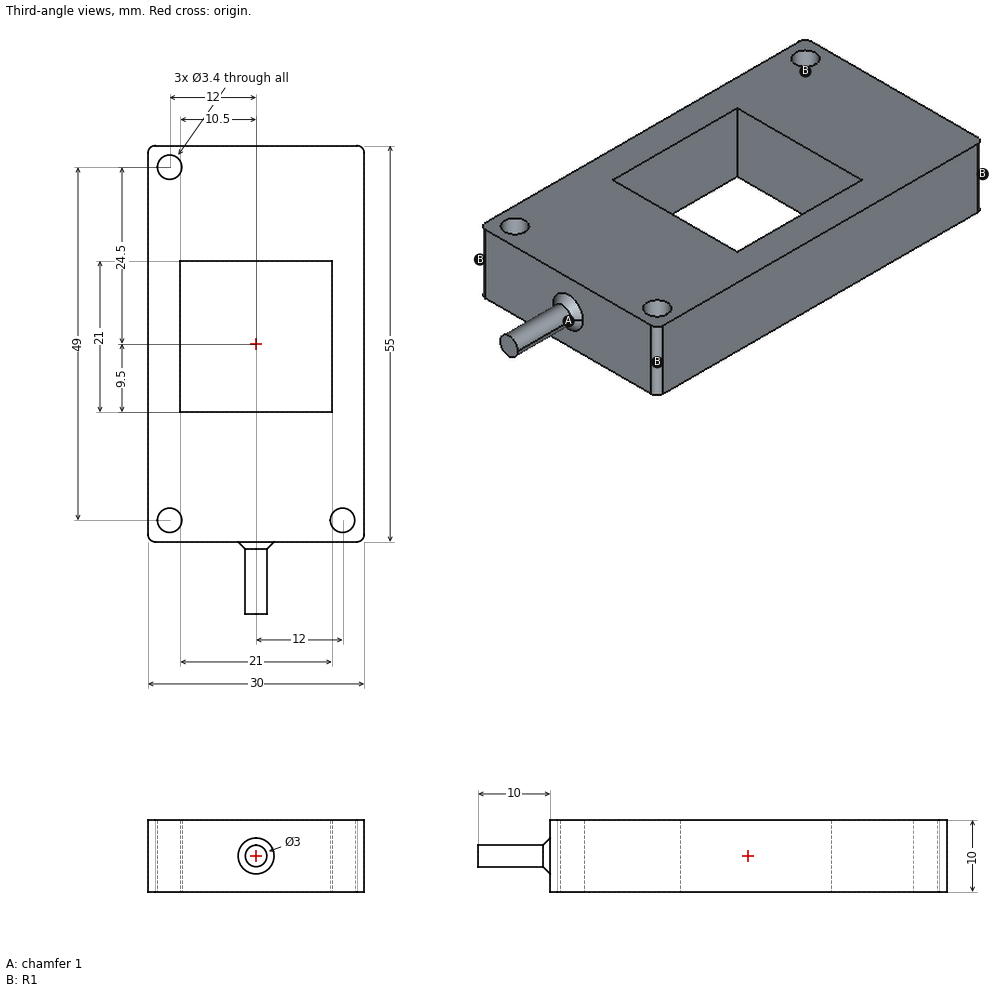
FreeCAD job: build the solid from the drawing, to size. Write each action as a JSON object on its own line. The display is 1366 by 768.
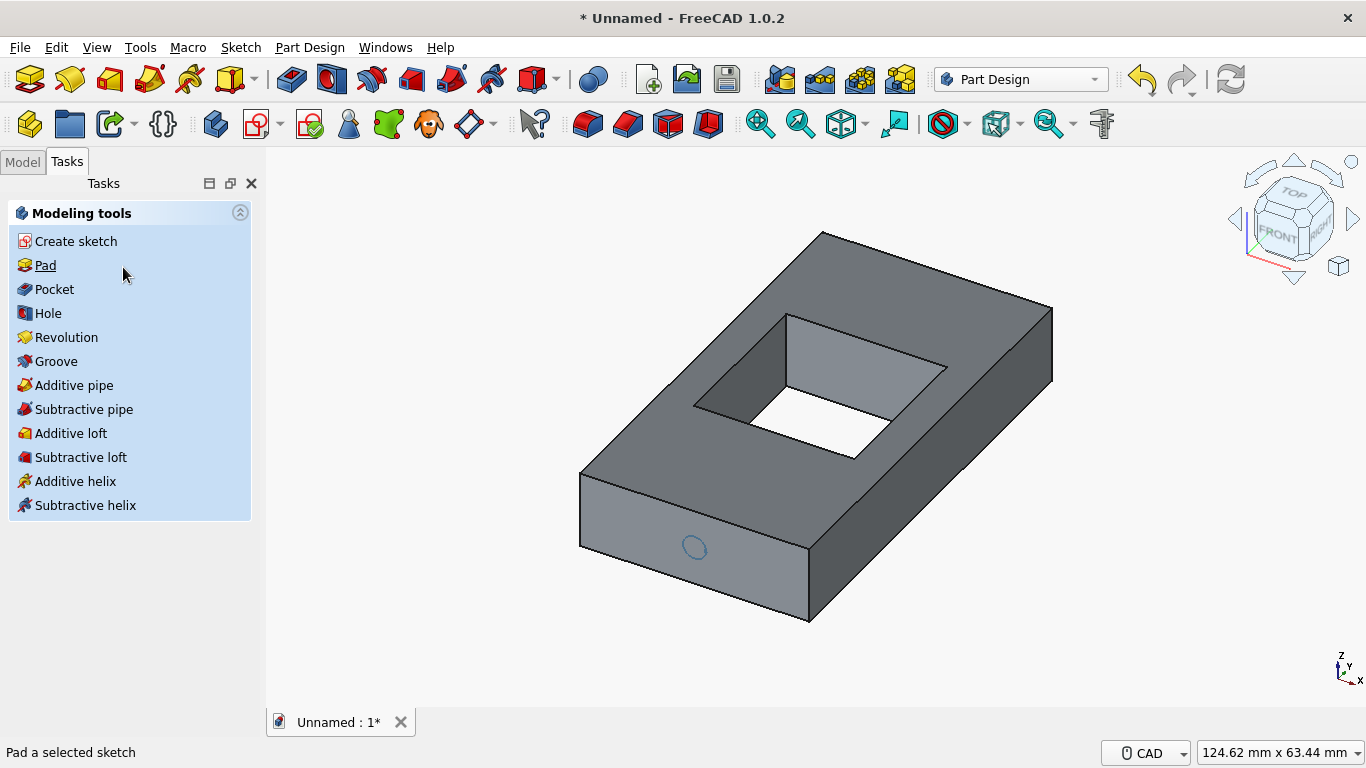
{"action": "left_click", "coordinate": [30, 80]}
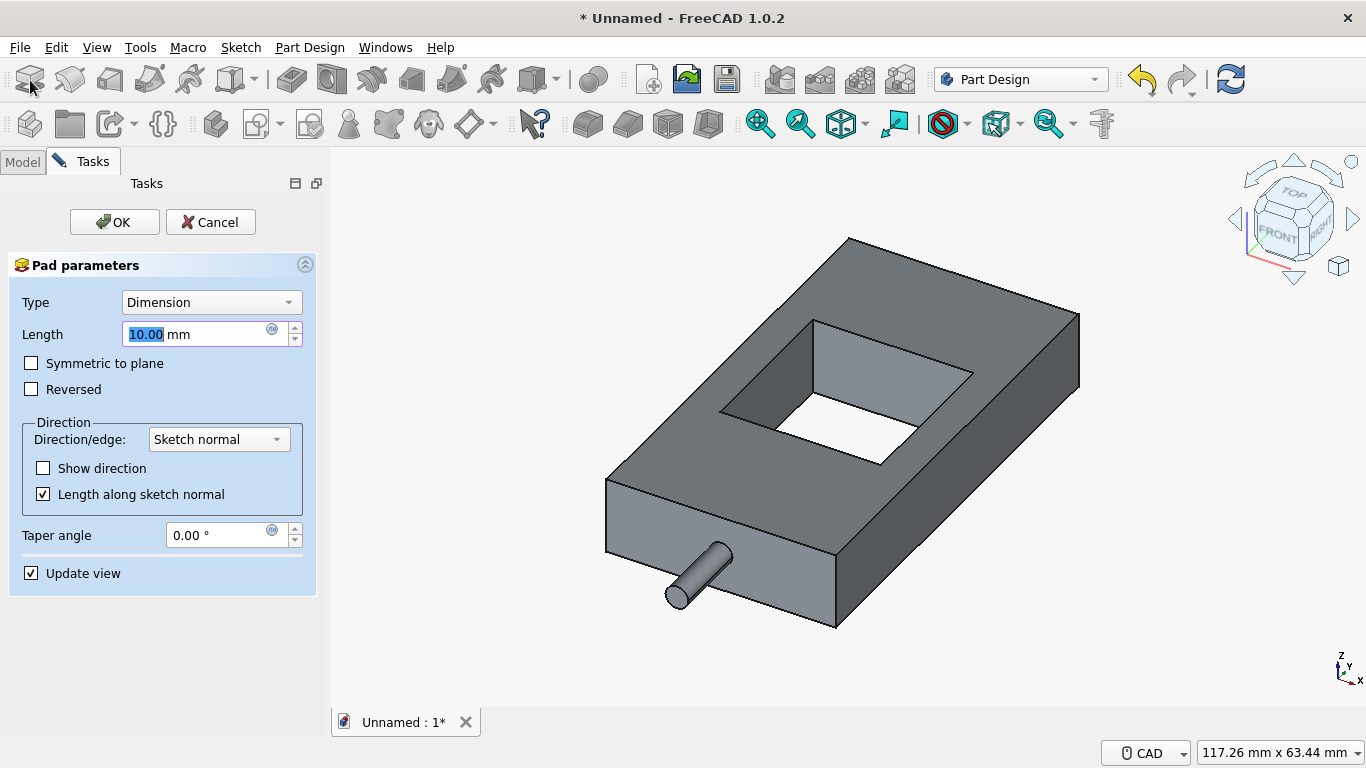
{"action": "type", "text": "10"}
{"action": "key", "text": "Tab"}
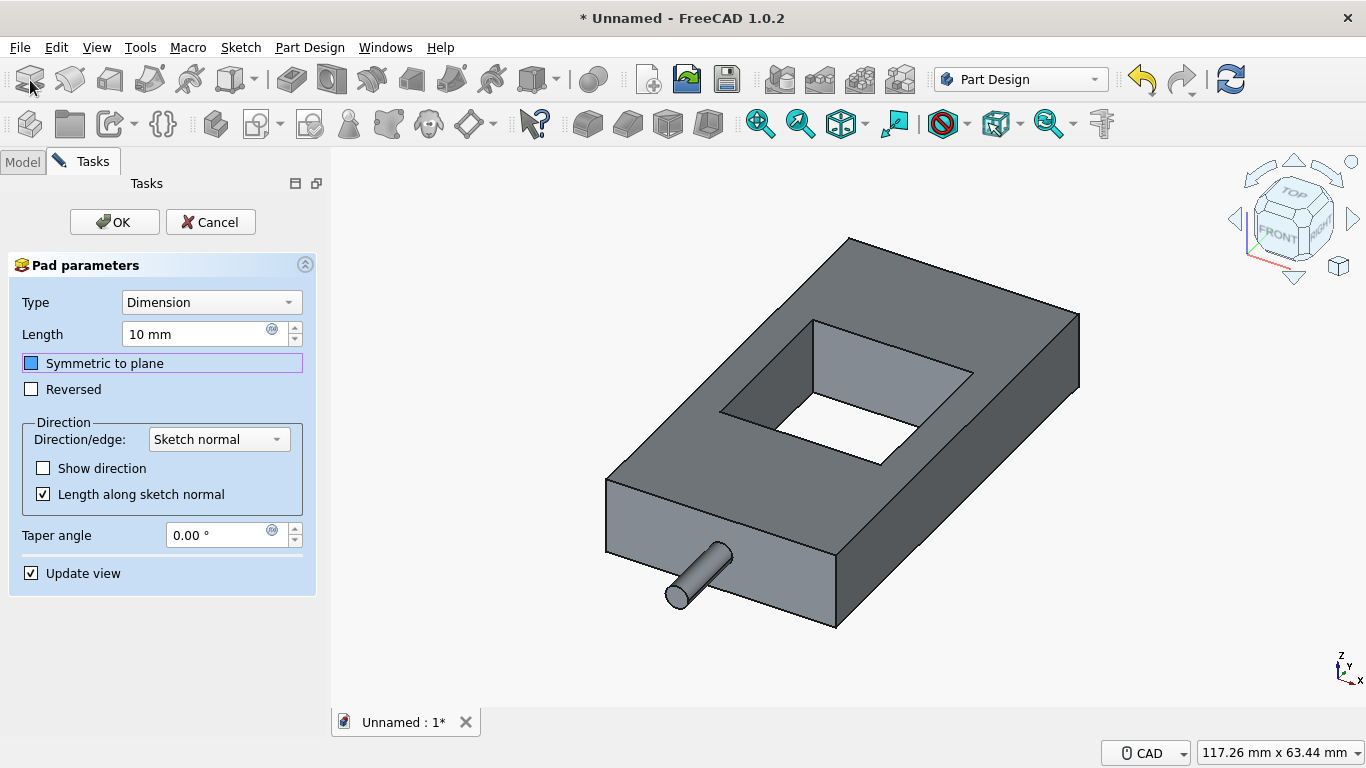
{"action": "left_click", "coordinate": [115, 222]}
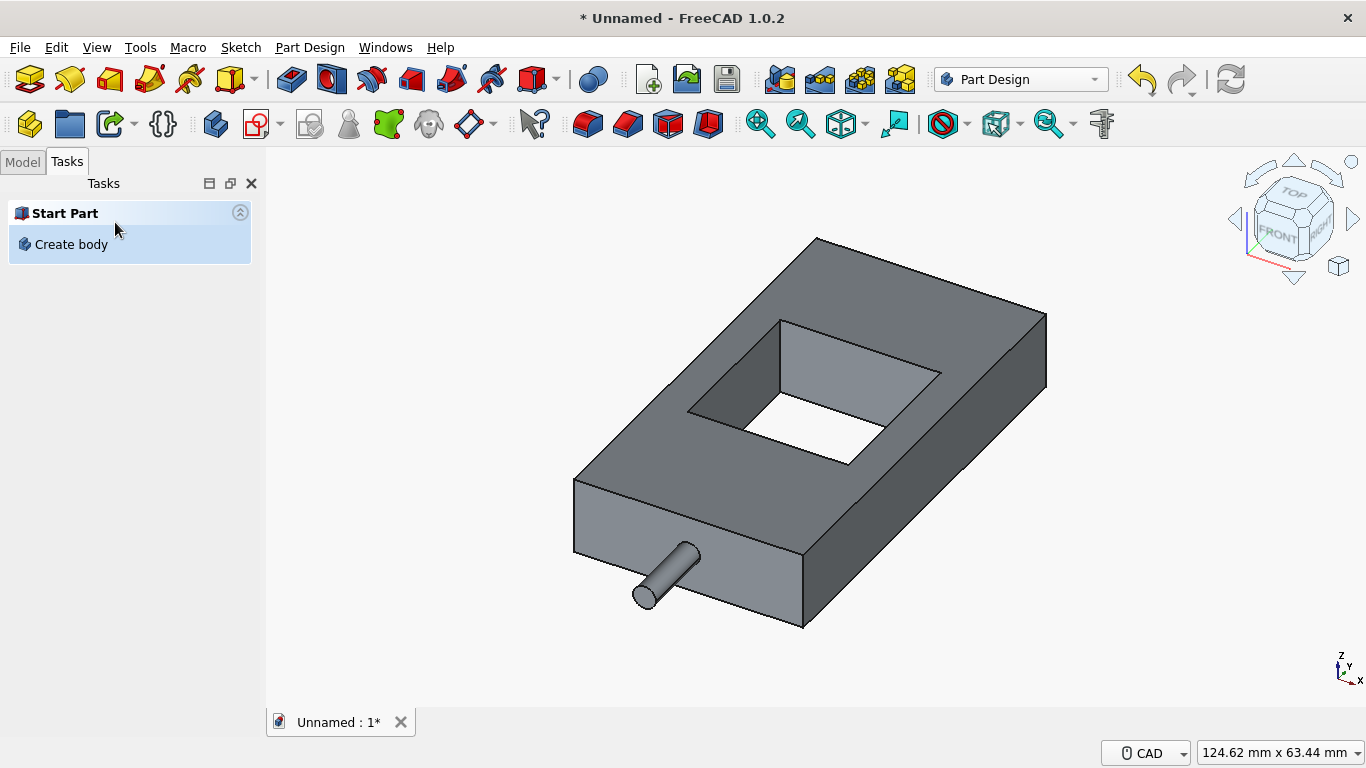
{"action": "left_click", "coordinate": [685, 541]}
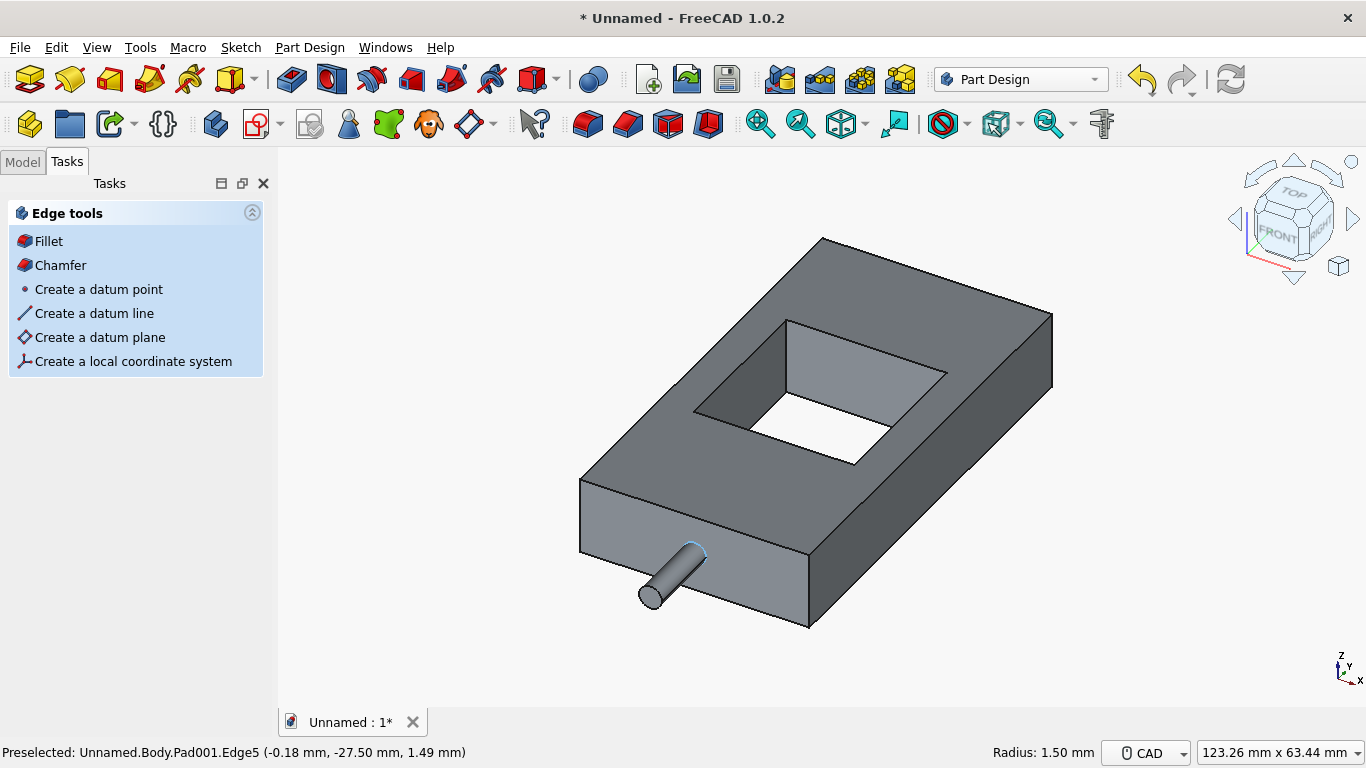
{"action": "left_click", "coordinate": [628, 124]}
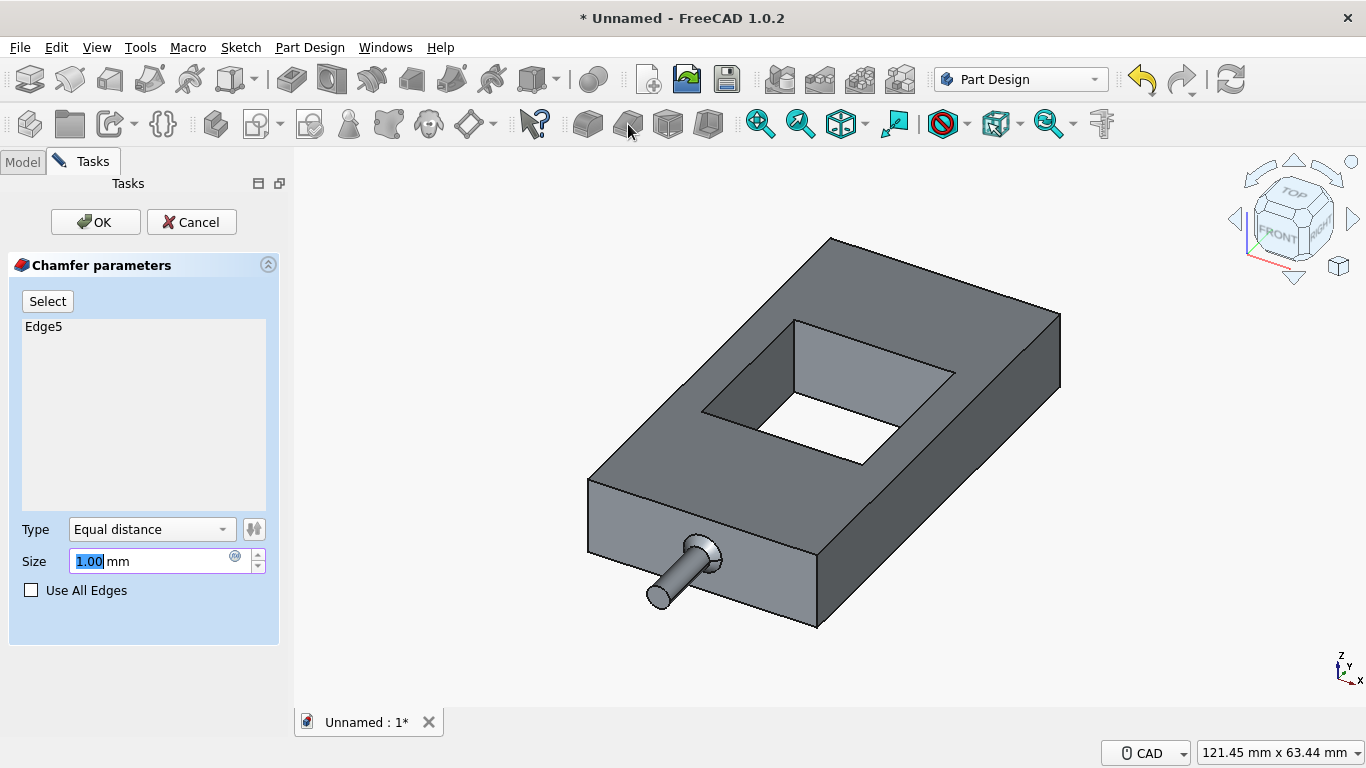
{"action": "type", "text": "1"}
{"action": "key", "text": "Tab"}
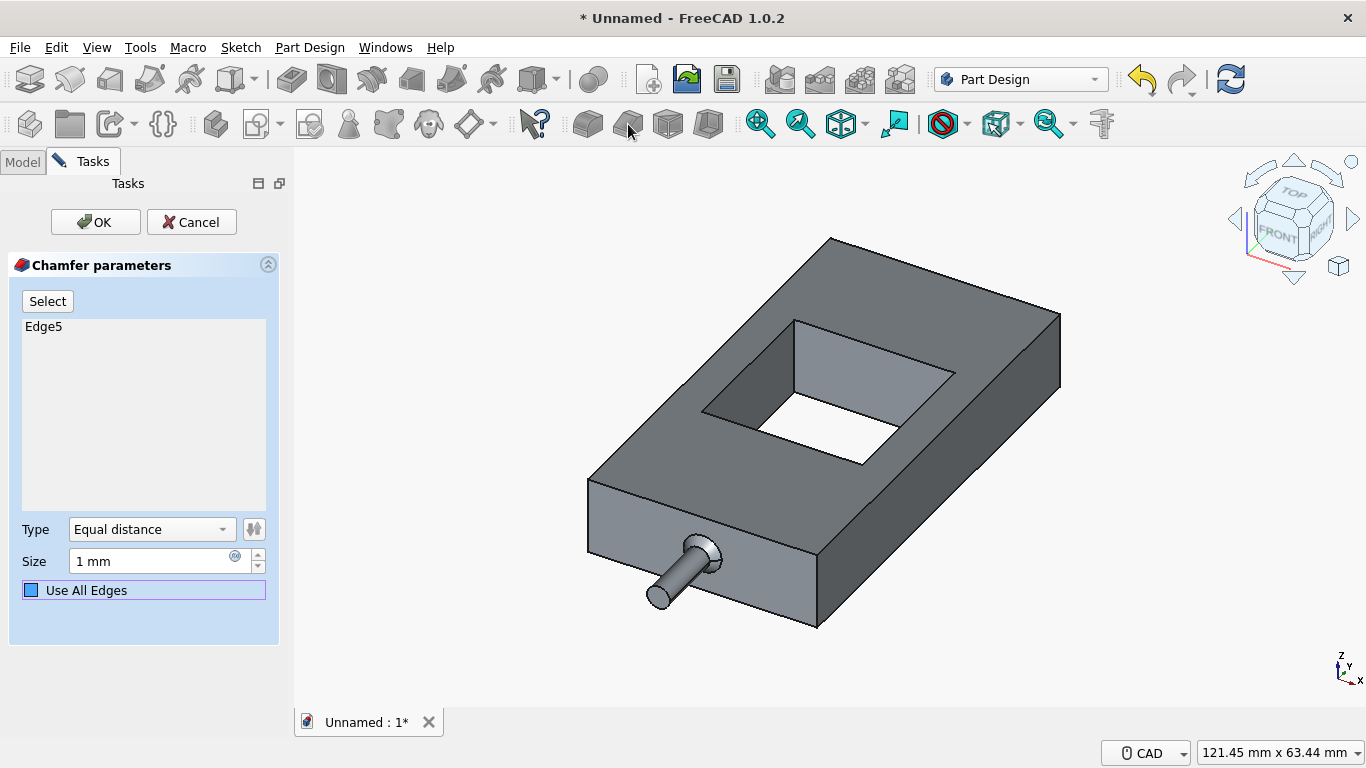
{"action": "left_click", "coordinate": [96, 222]}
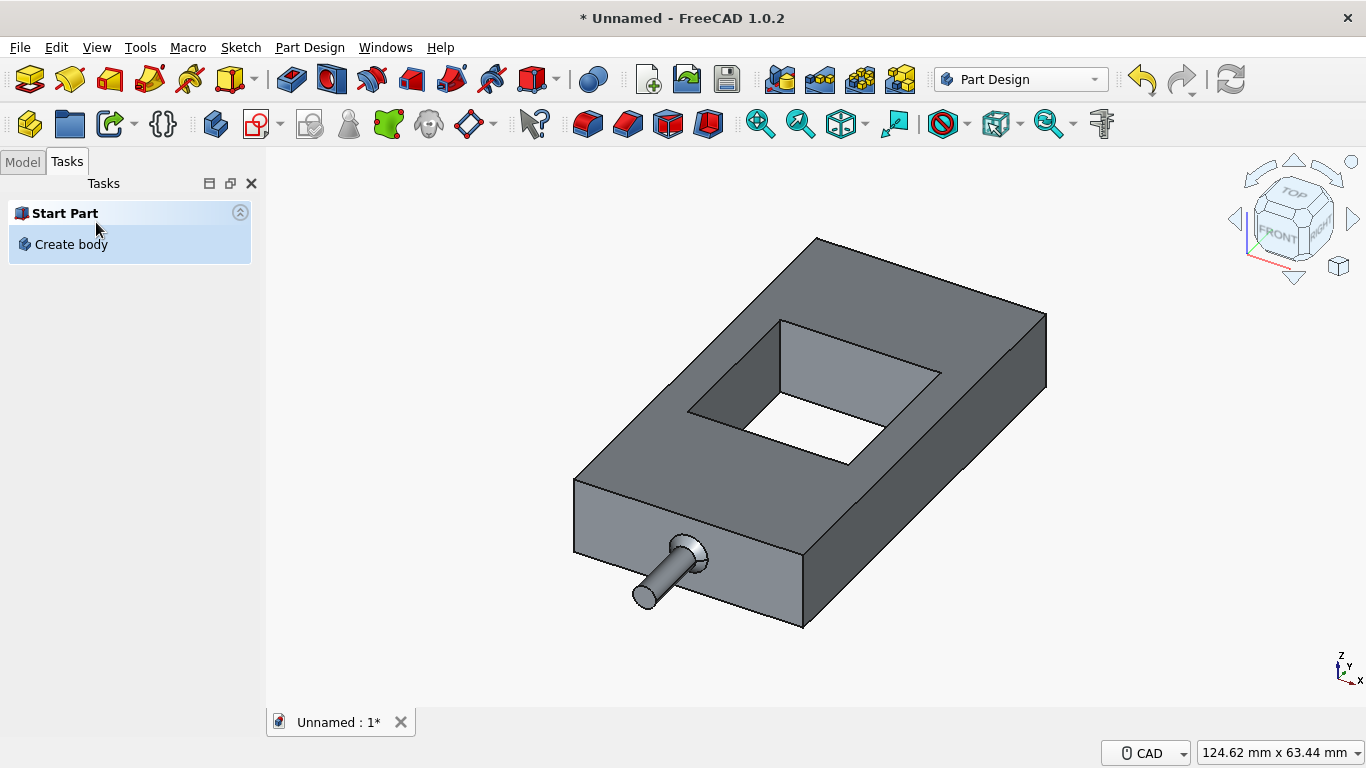
{"action": "left_click", "coordinate": [803, 591]}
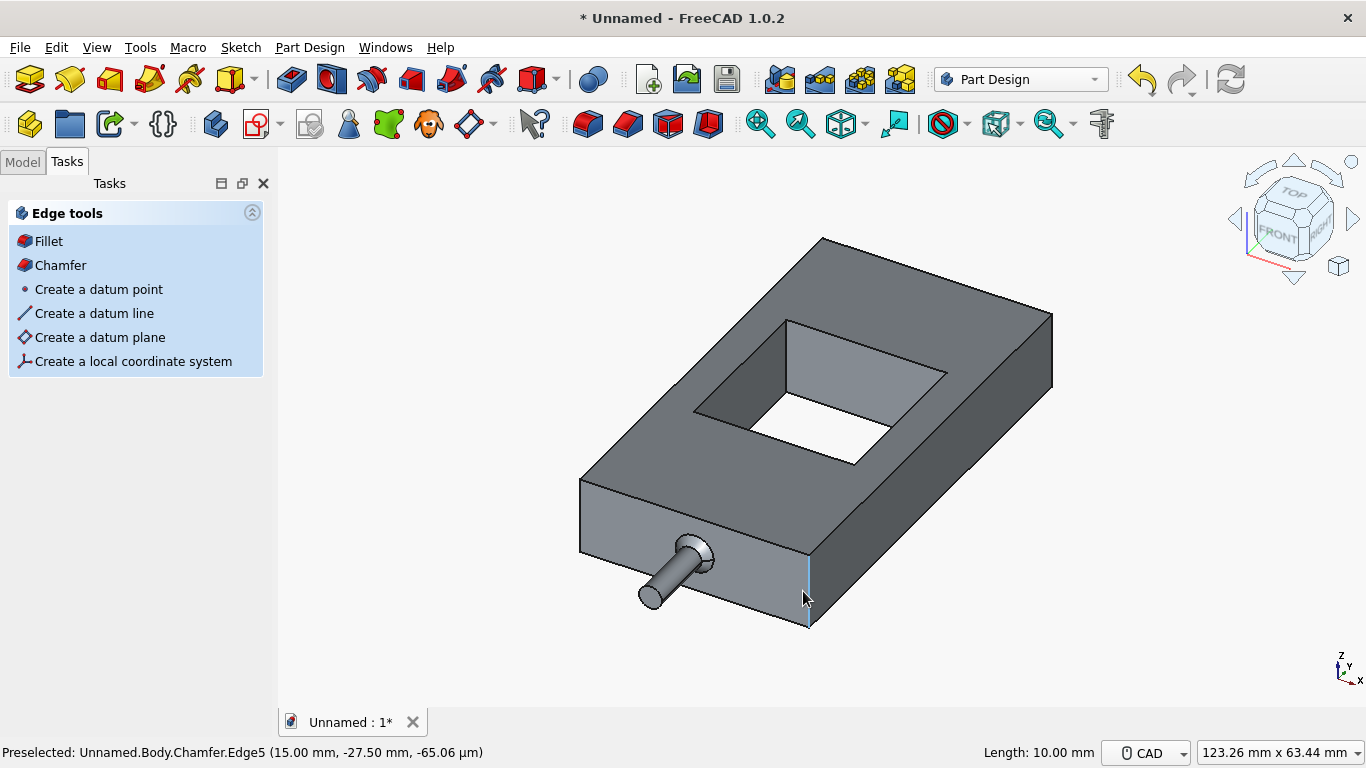
{"action": "key", "text": "0"}